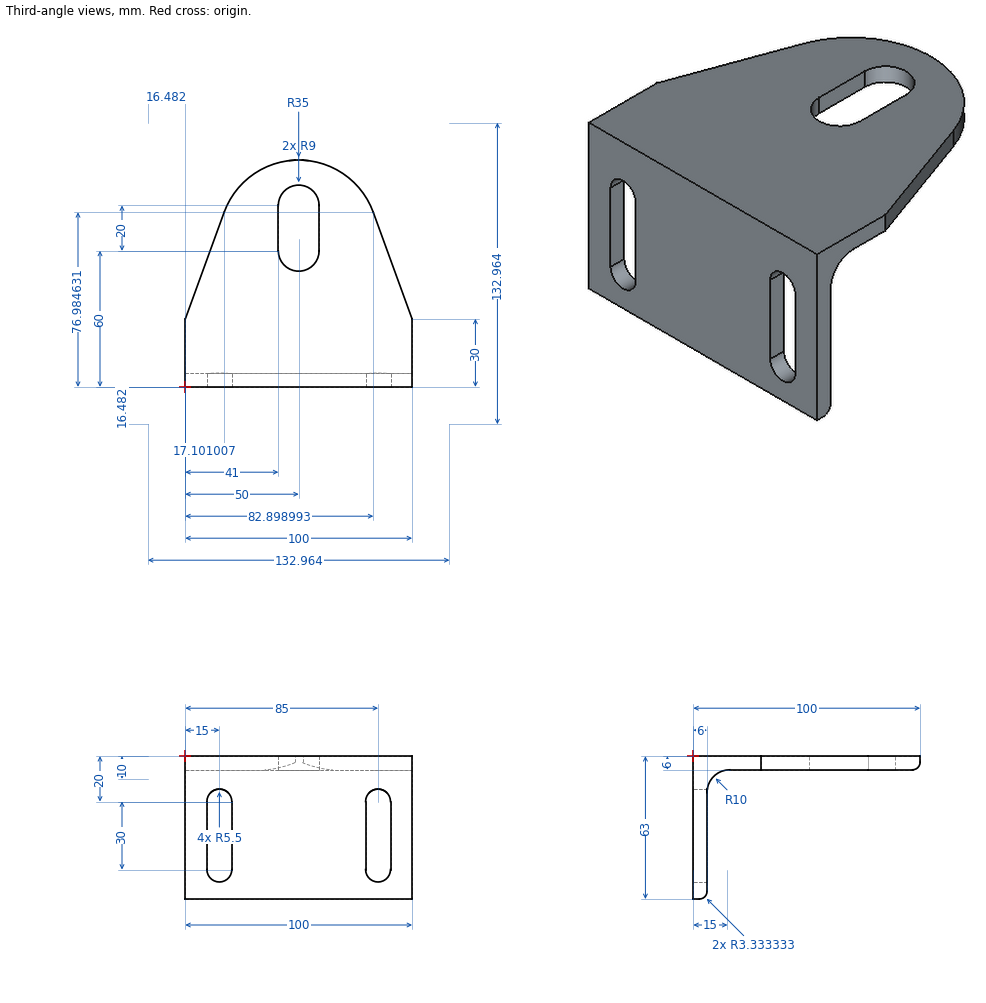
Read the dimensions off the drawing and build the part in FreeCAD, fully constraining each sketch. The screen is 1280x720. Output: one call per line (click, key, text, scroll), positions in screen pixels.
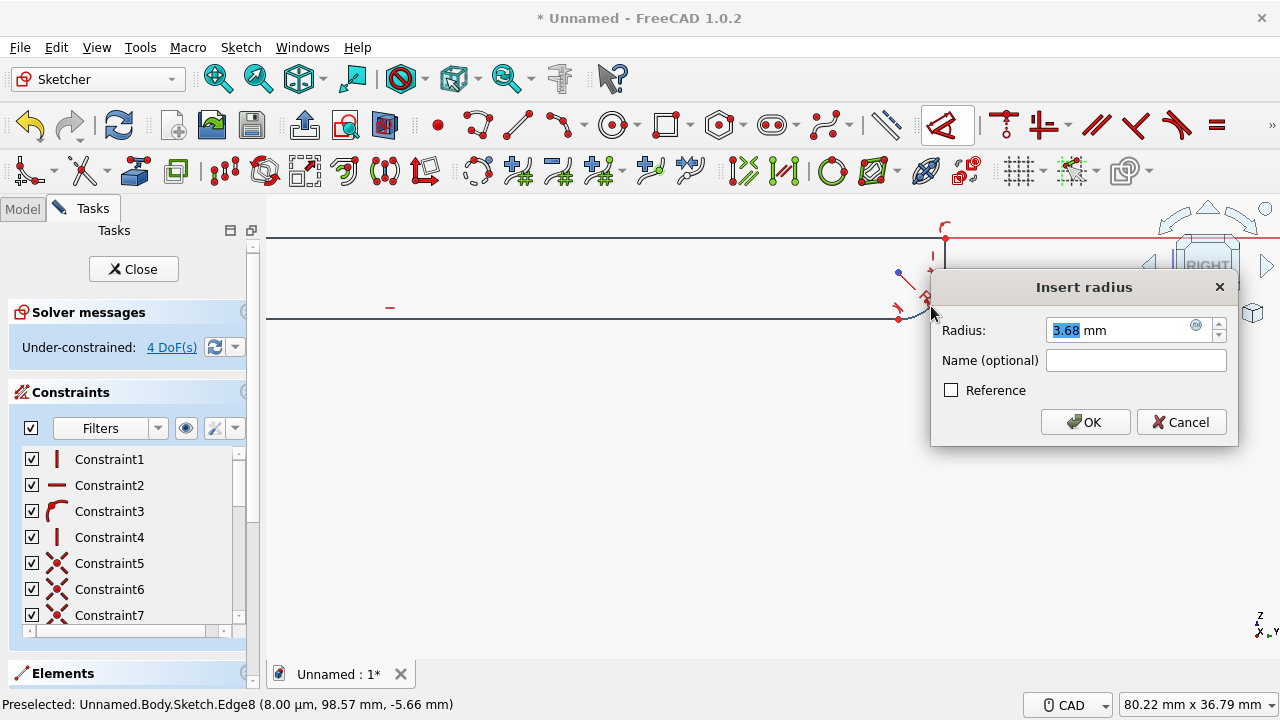
text(3.333333)
key(Return)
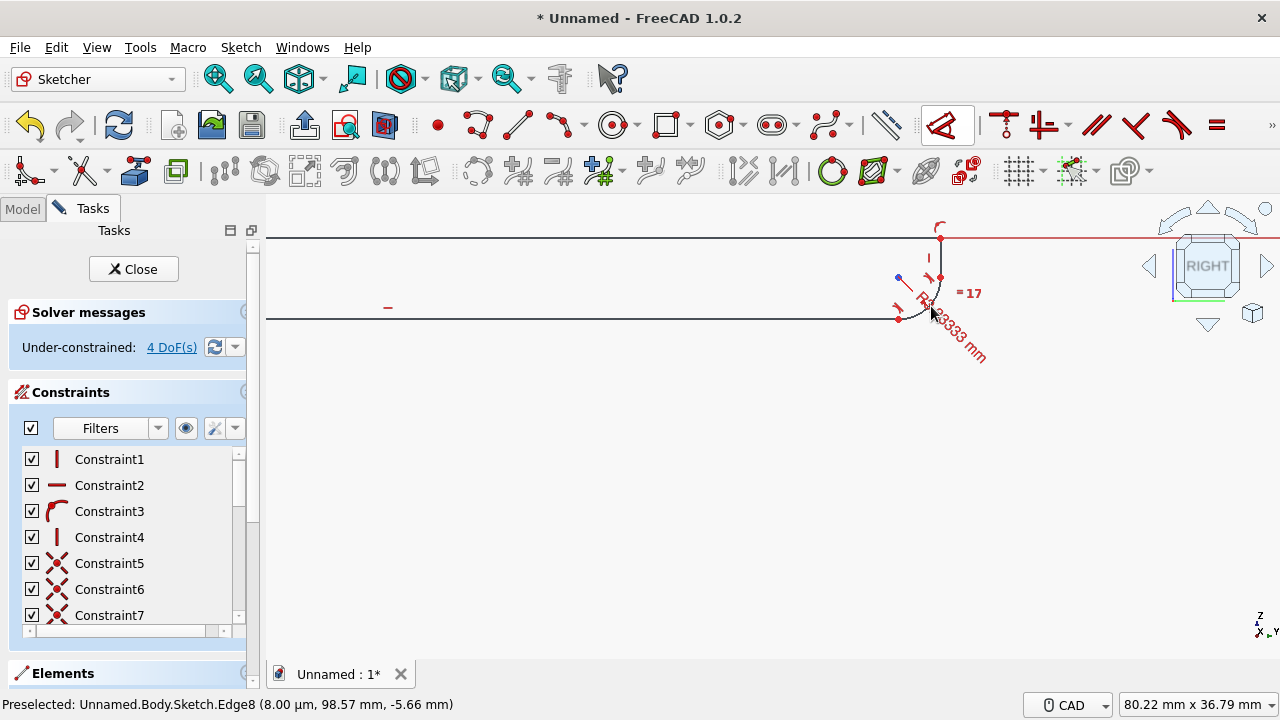
scroll(932, 304, down, 5)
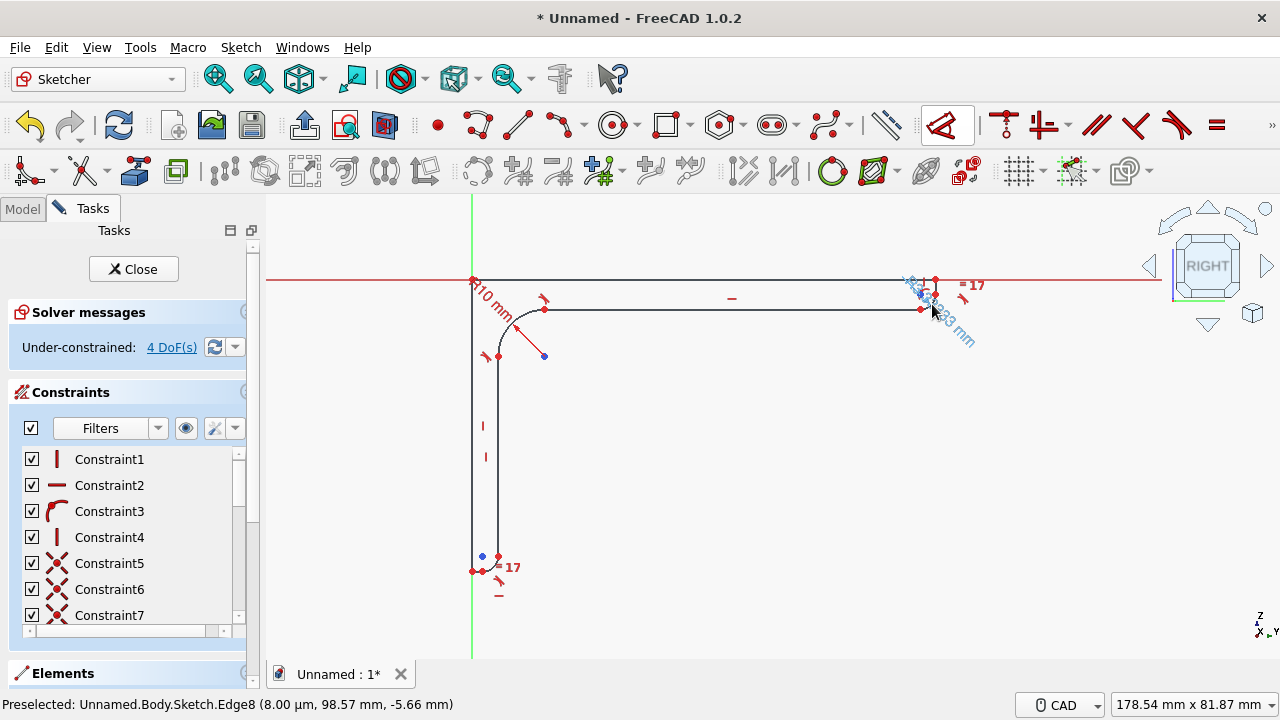
click(472, 367)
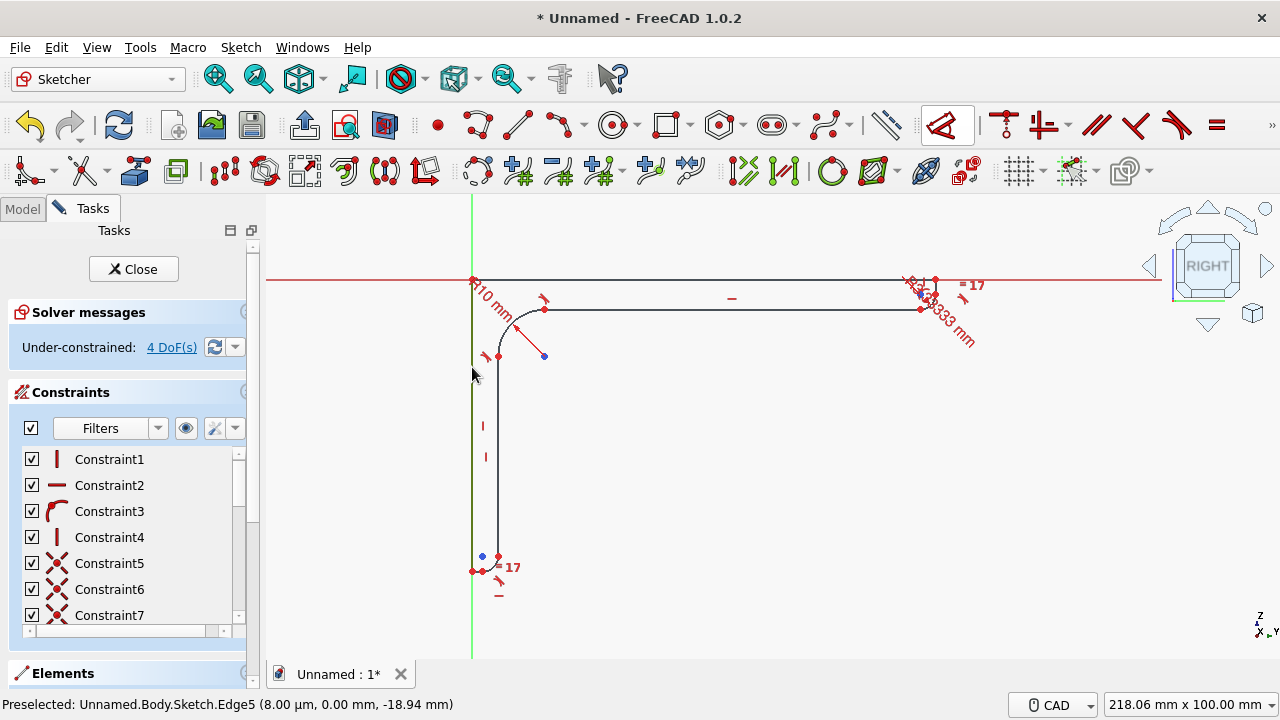
click(968, 126)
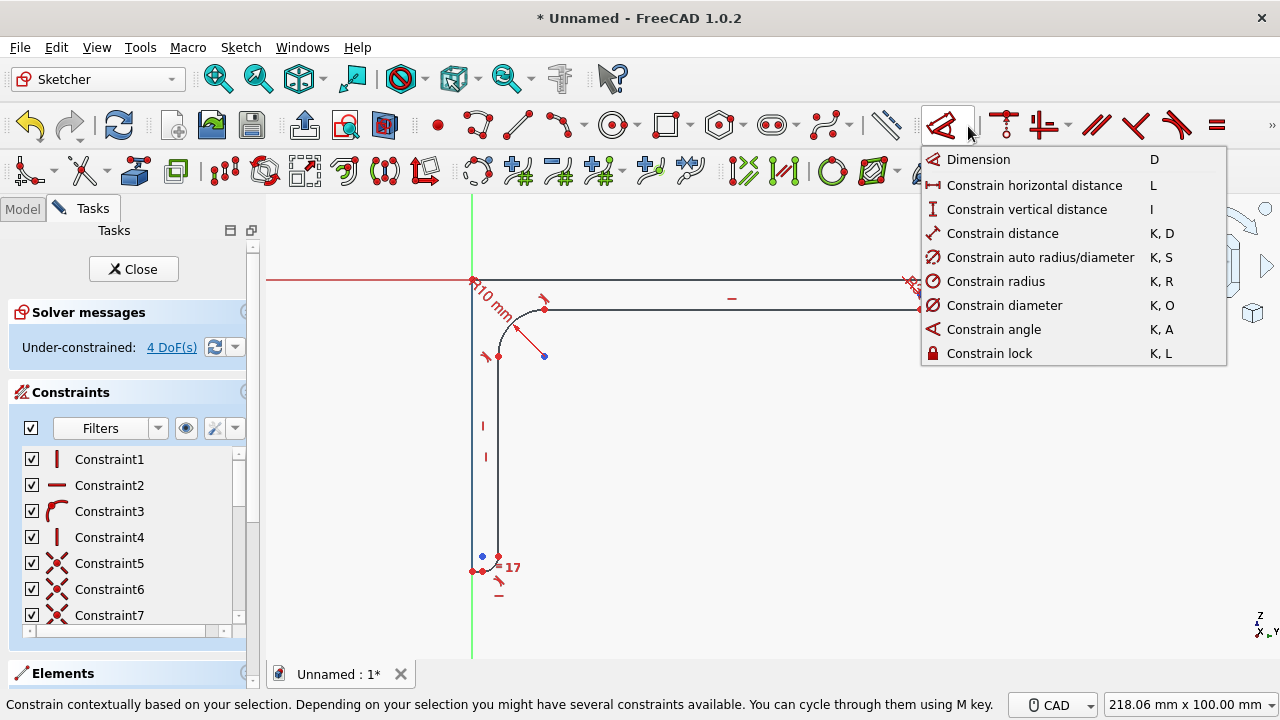
click(1074, 209)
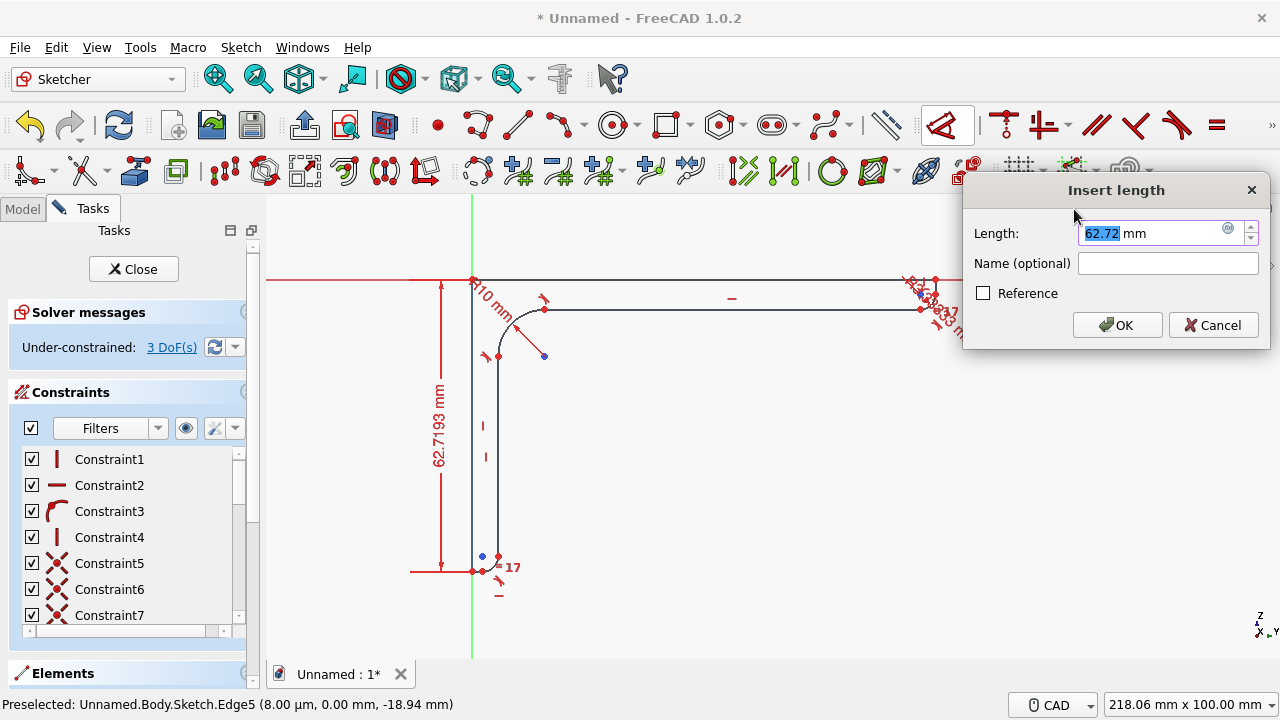
text(63)
key(Return)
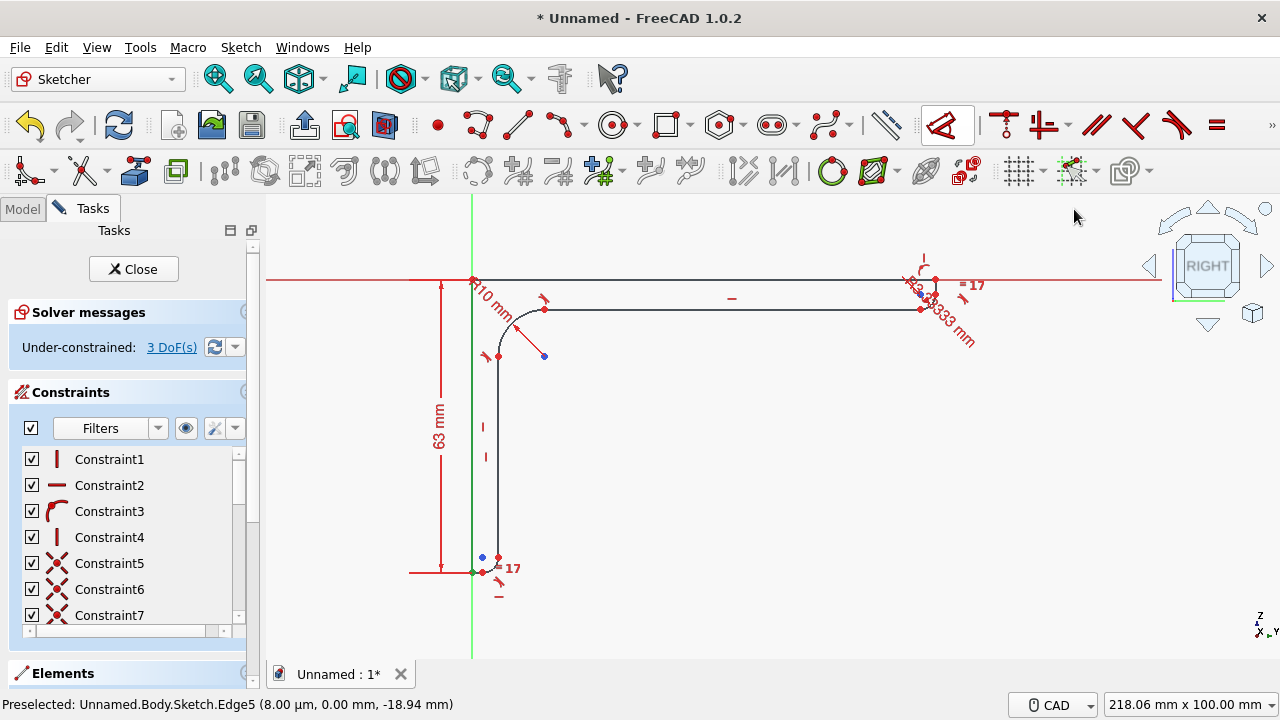
scroll(498, 557, up, 2)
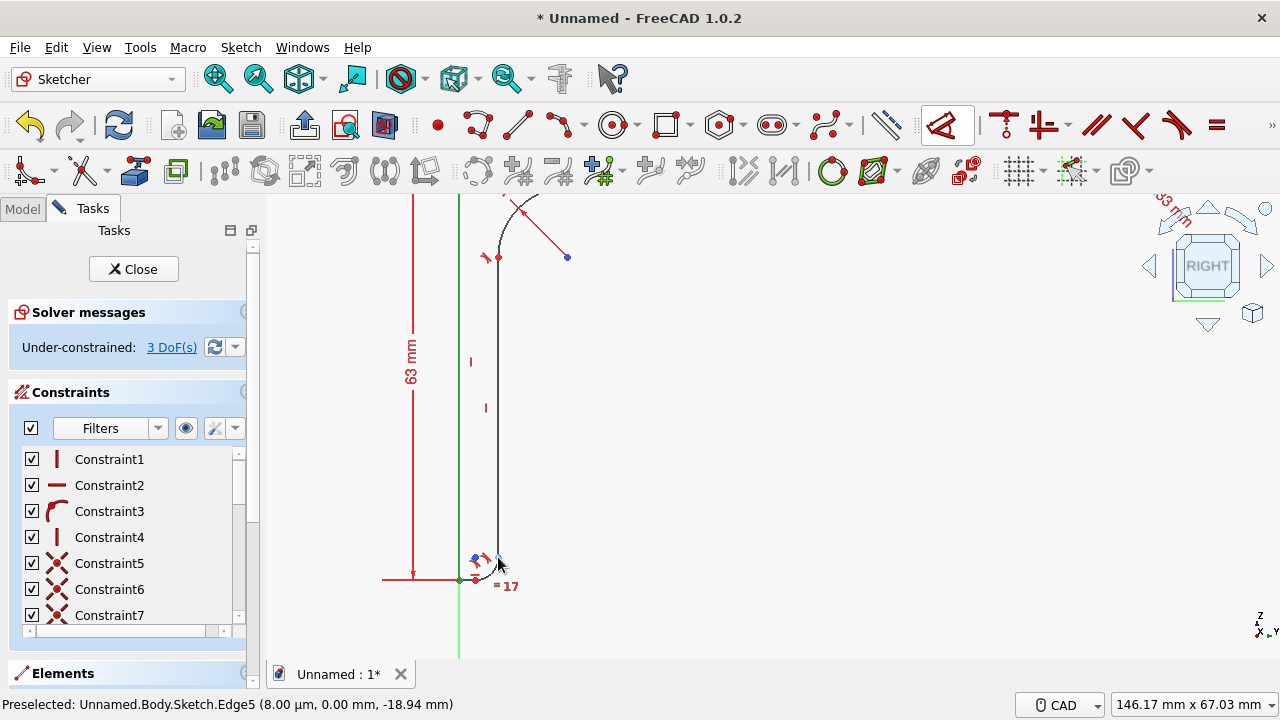
click(498, 557)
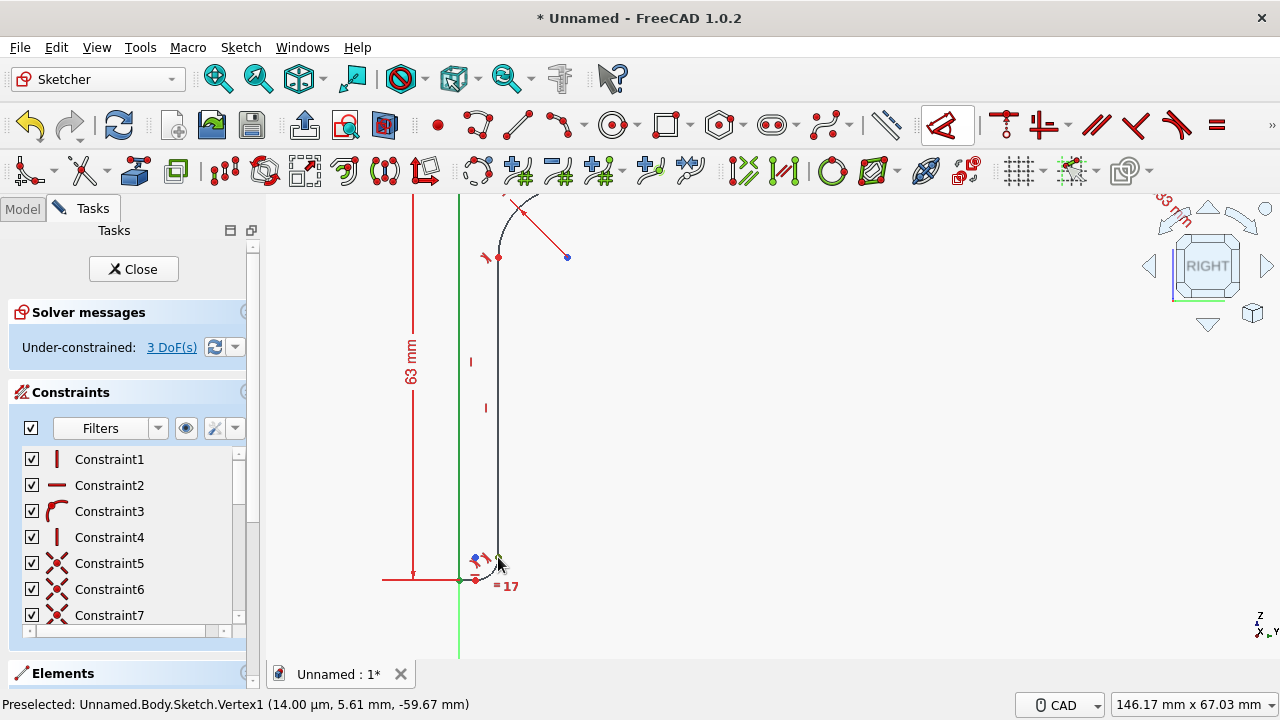
key(l)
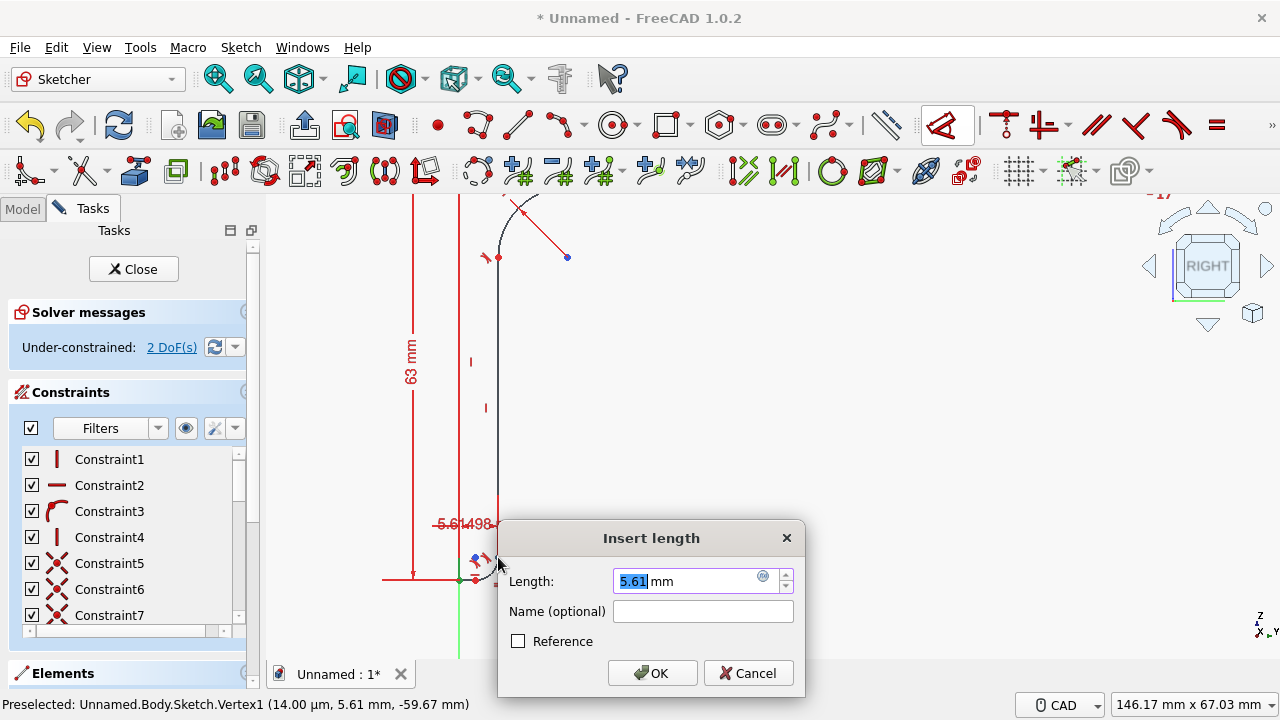
text(6)
key(Return)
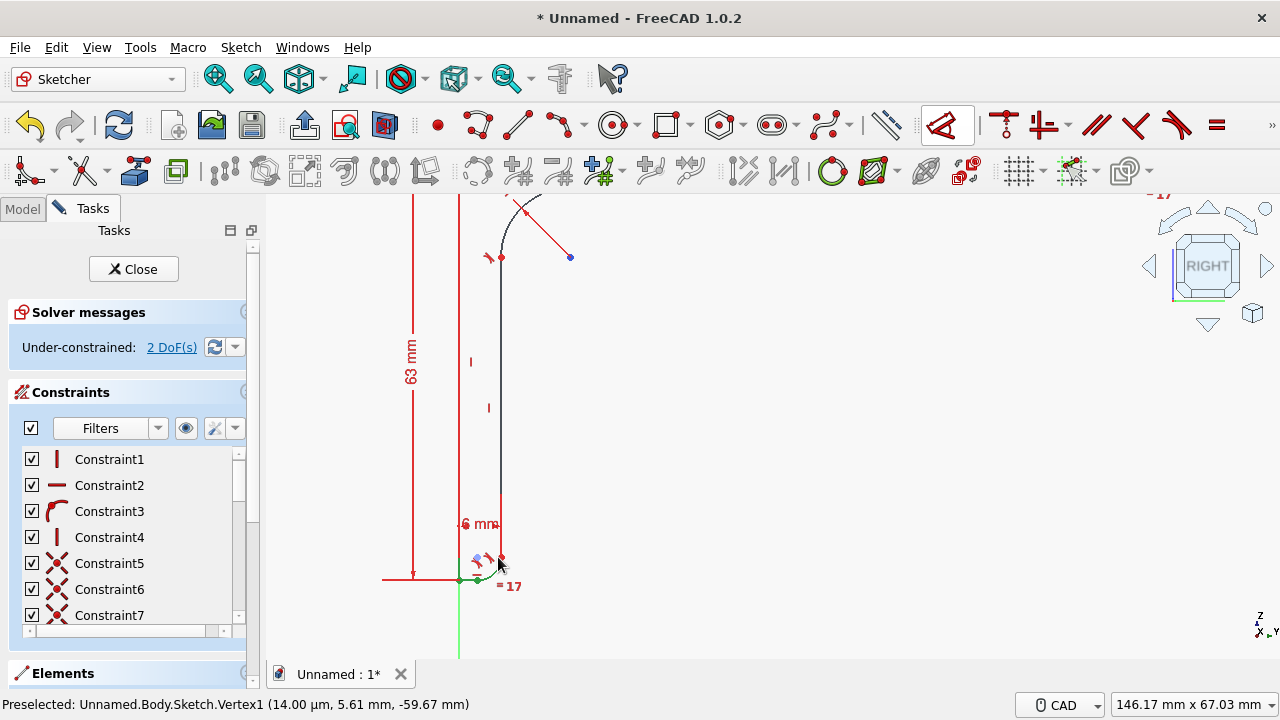
scroll(498, 558, down, 2)